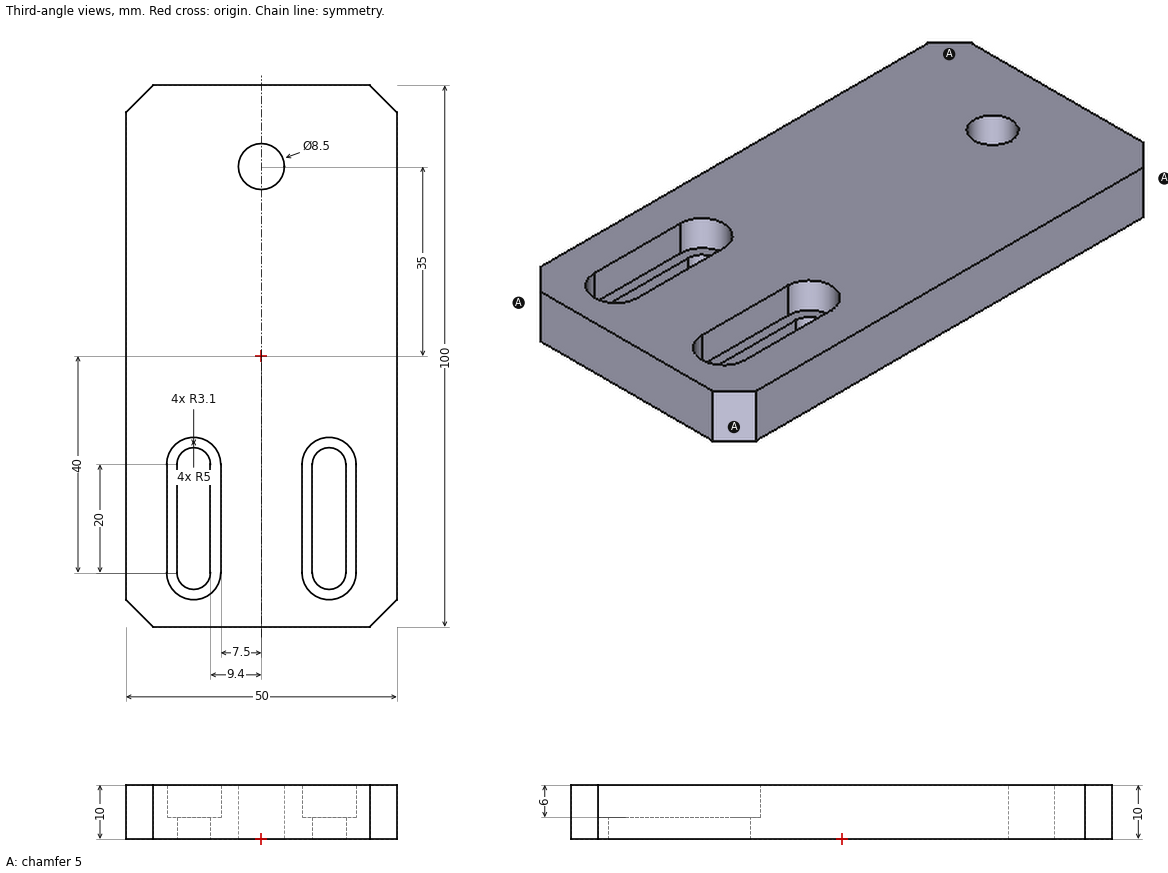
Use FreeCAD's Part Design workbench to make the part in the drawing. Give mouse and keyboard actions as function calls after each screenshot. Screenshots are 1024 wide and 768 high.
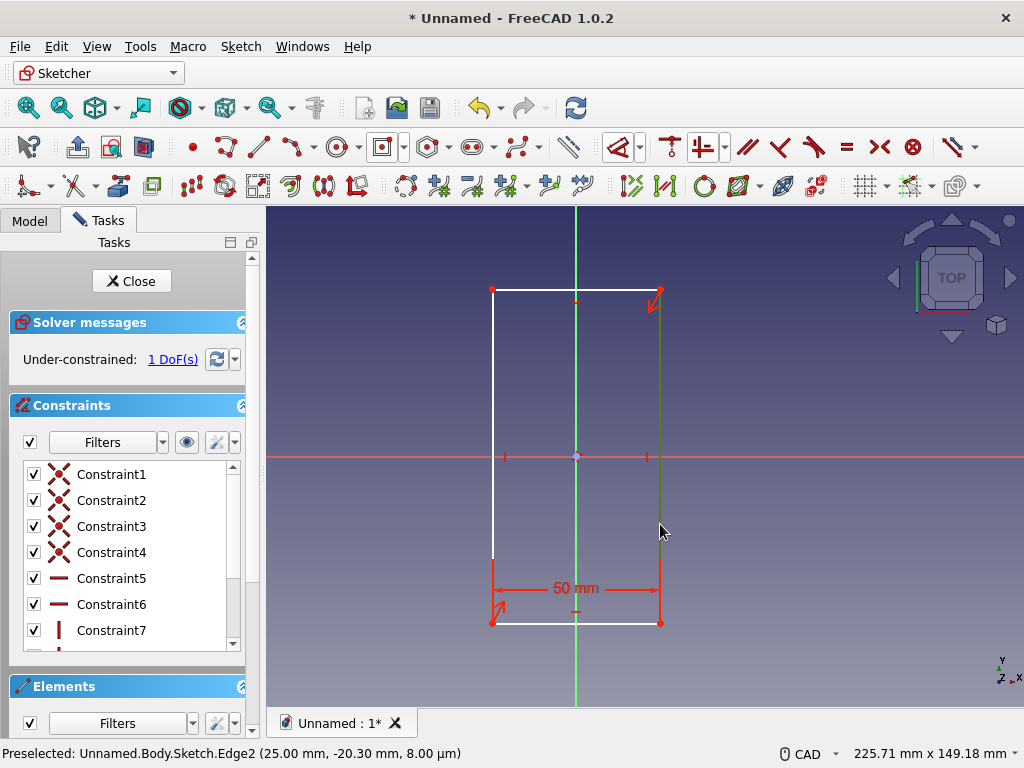
key(i)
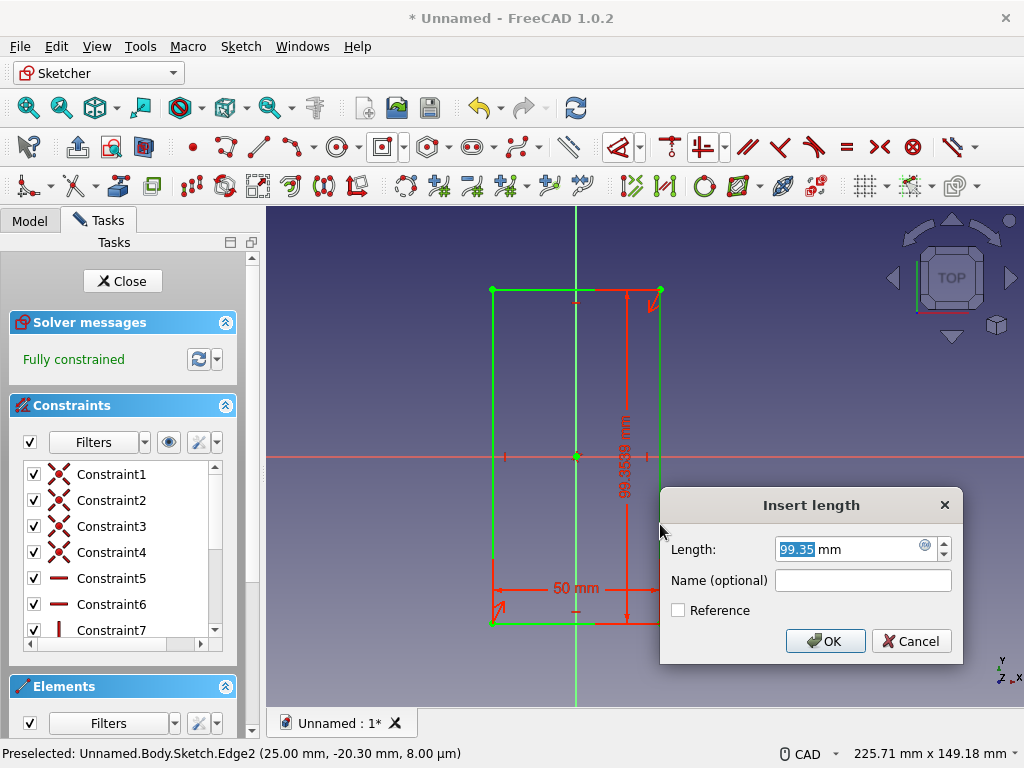
text(100)
key(Return)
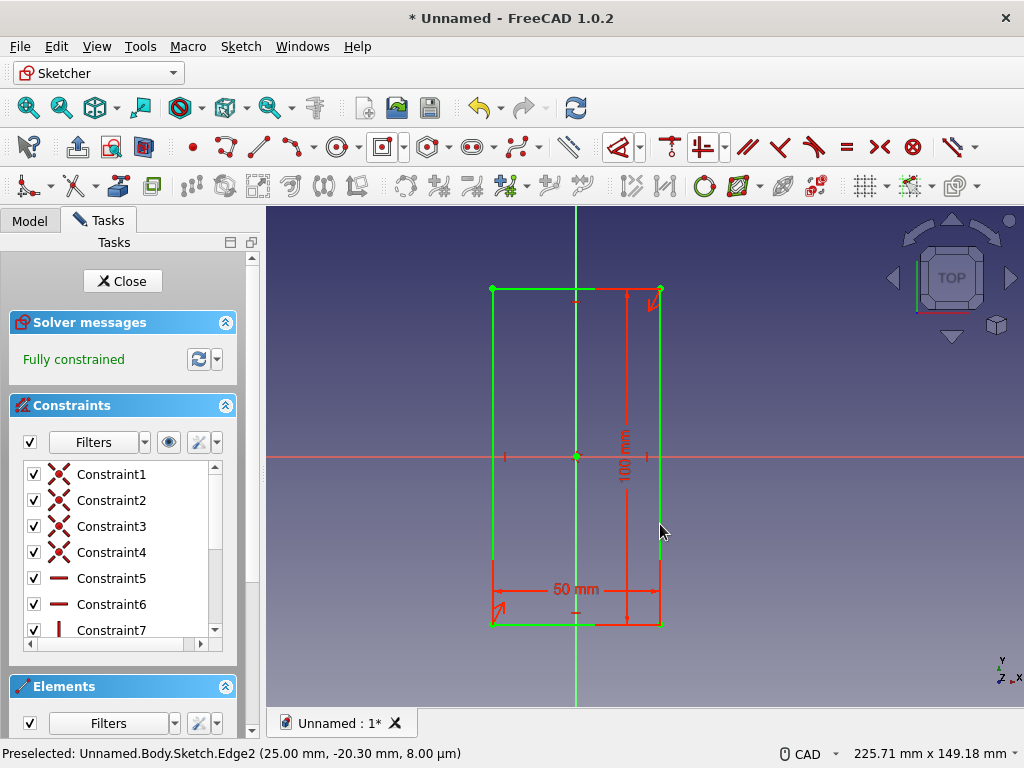
click(123, 281)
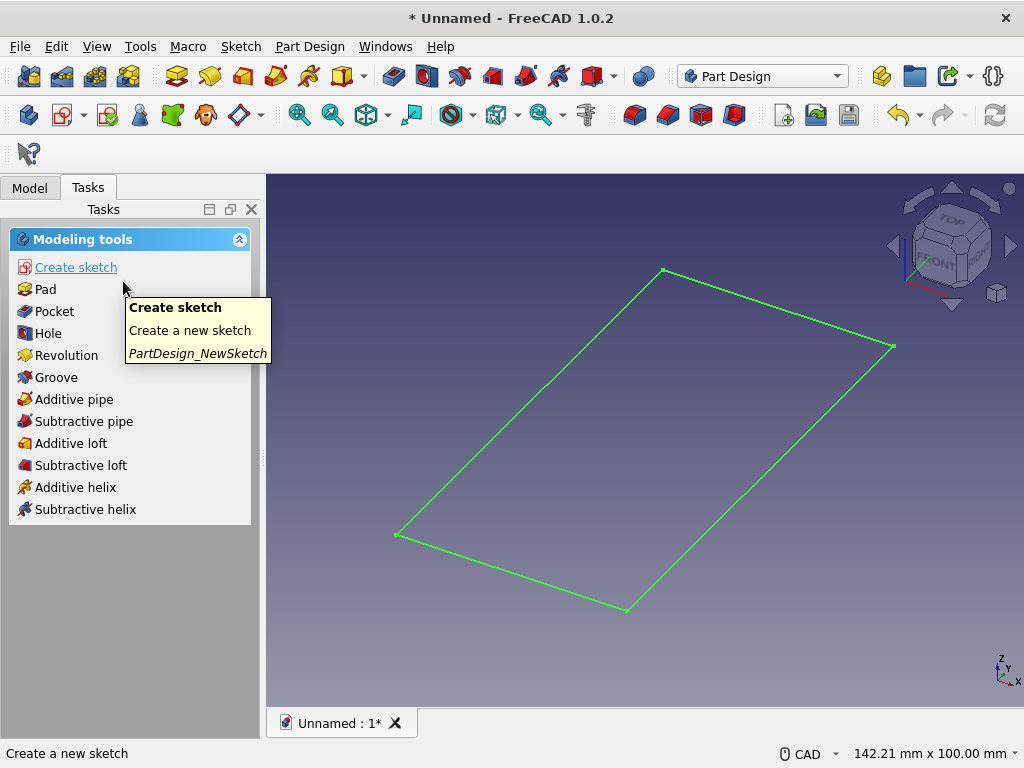
click(177, 76)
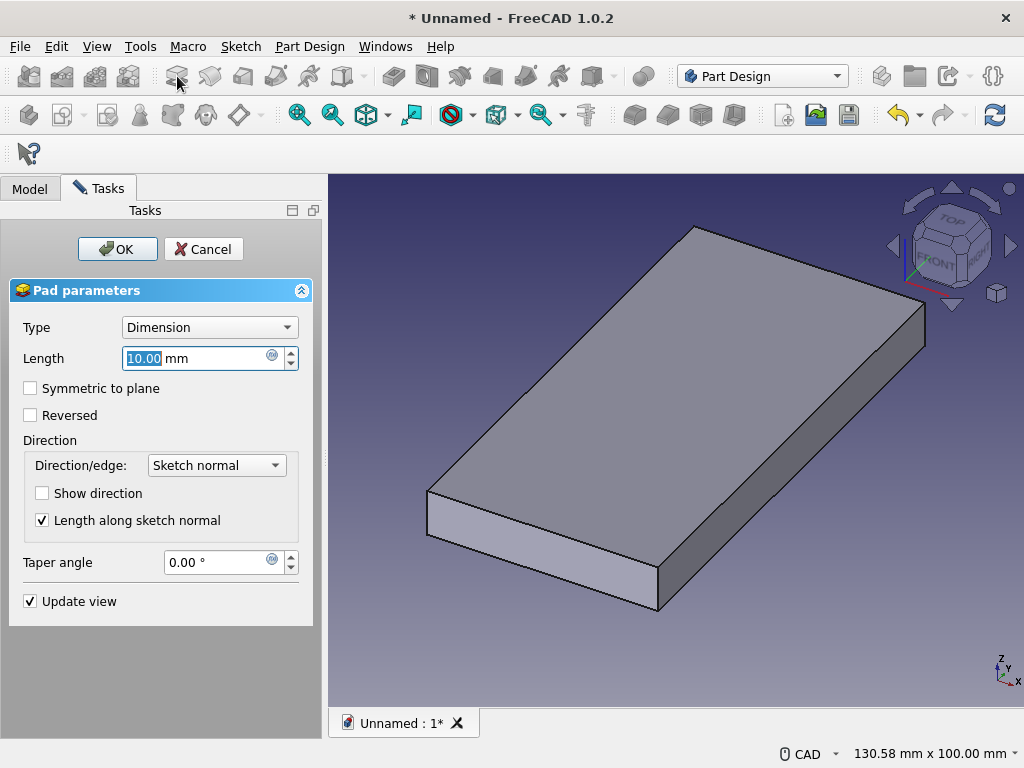
text(10)
key(Tab)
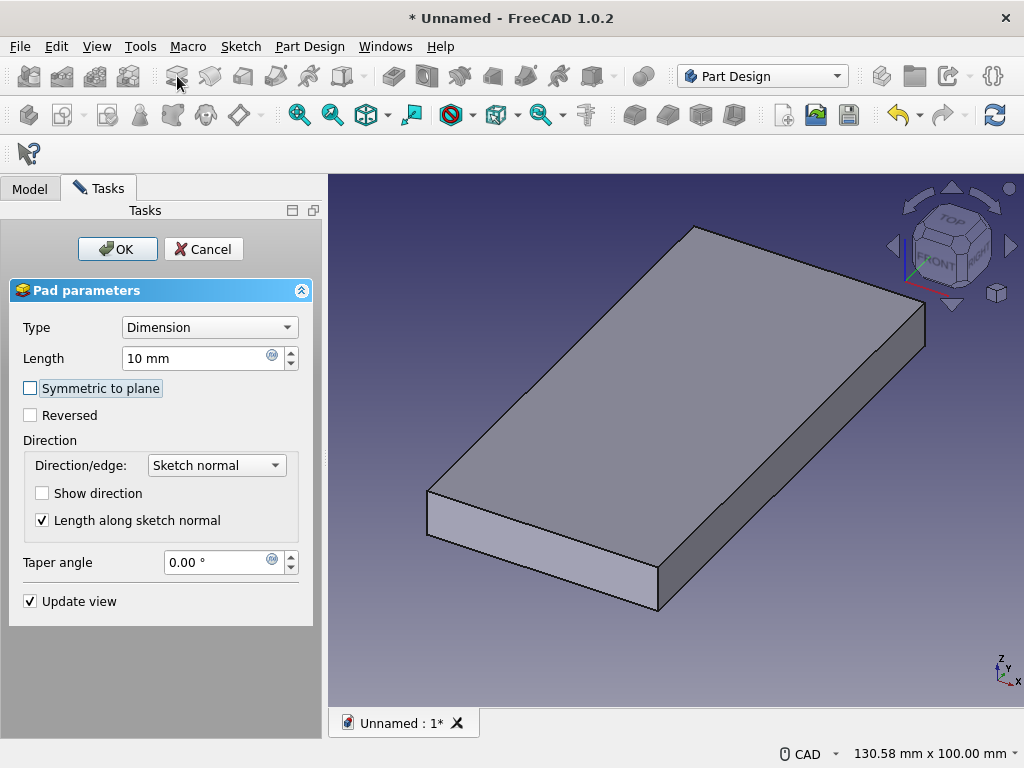
click(118, 249)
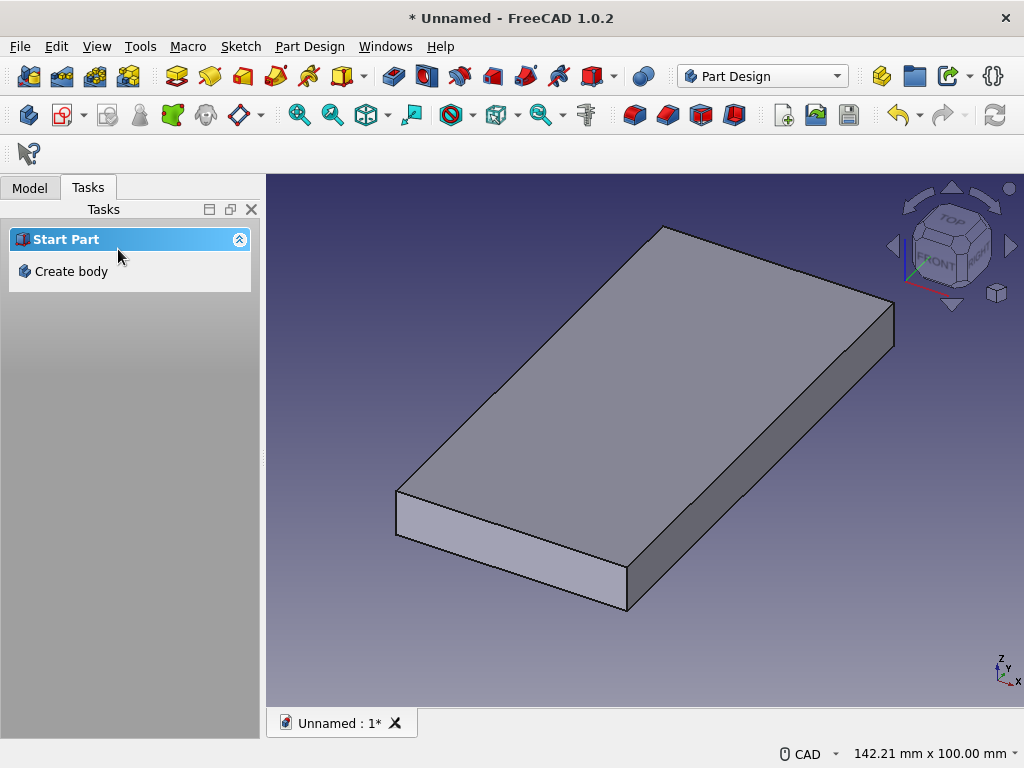
click(683, 358)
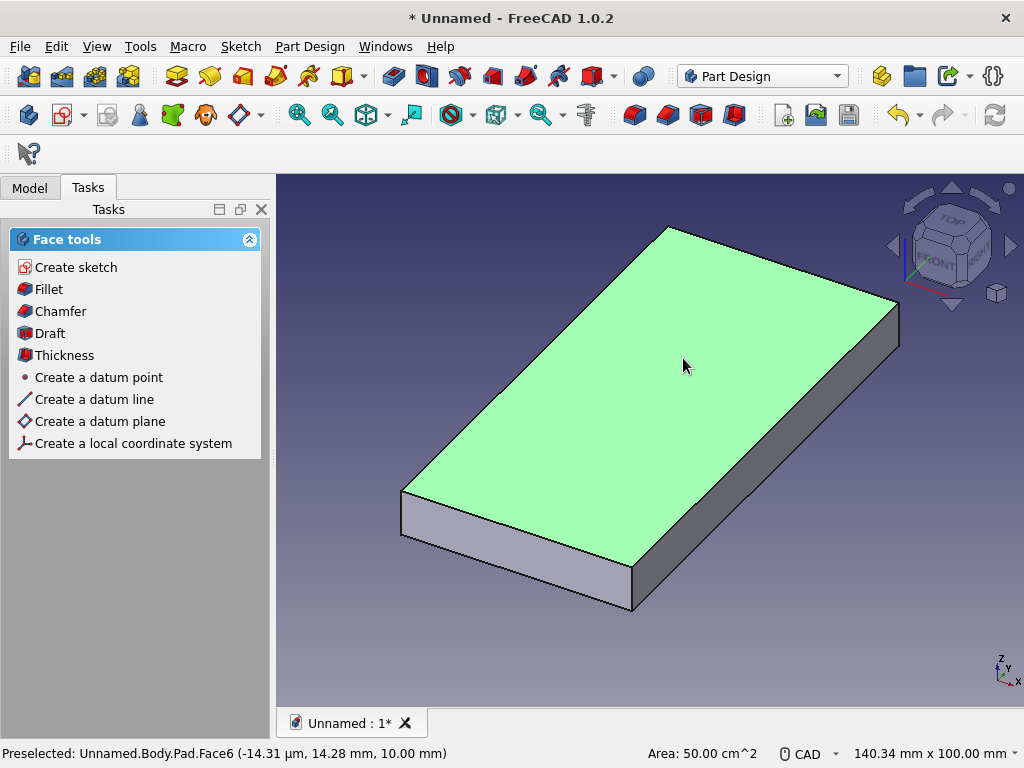
click(62, 116)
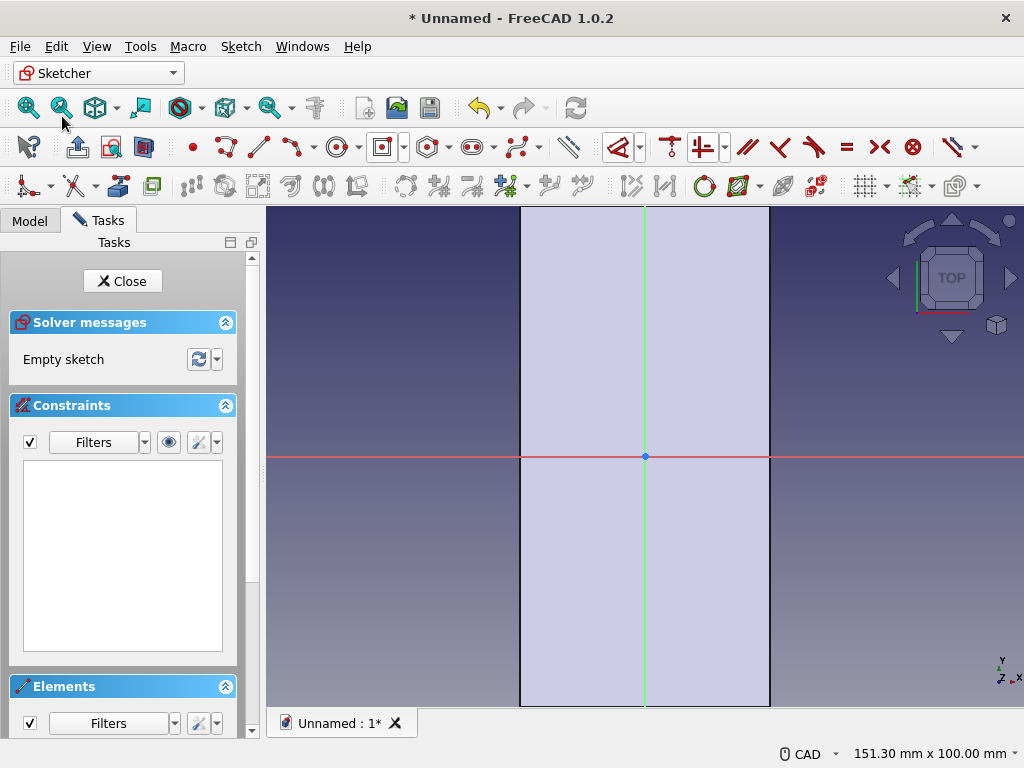
scroll(294, 234, down, 1)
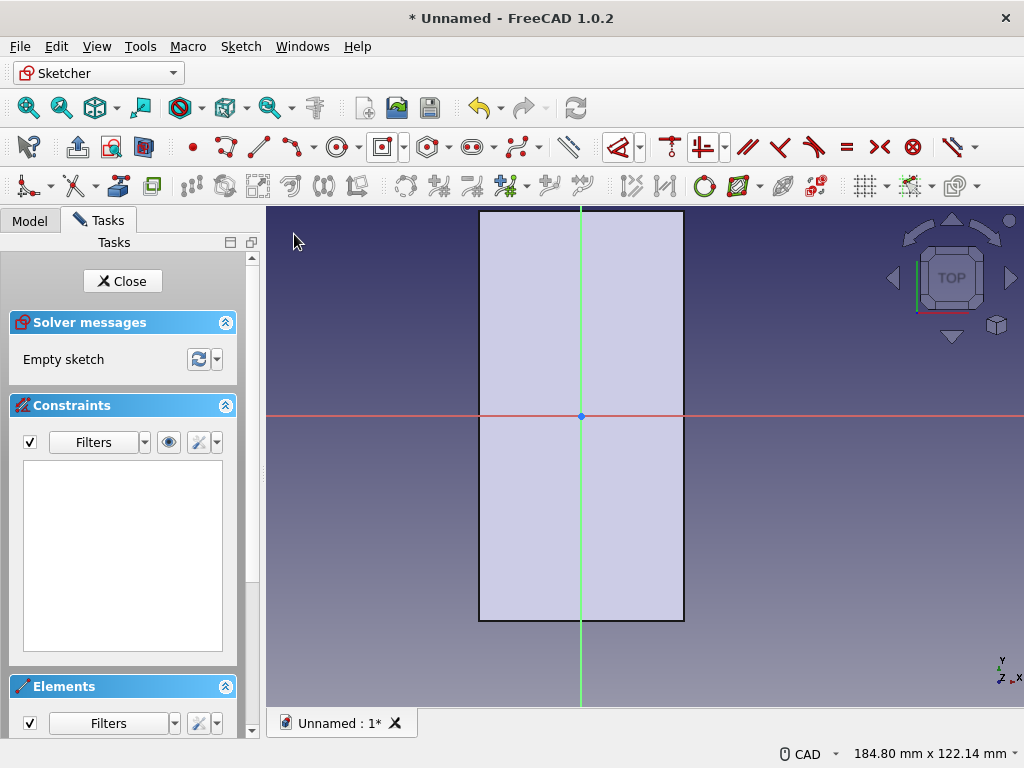
scroll(587, 563, up, 3)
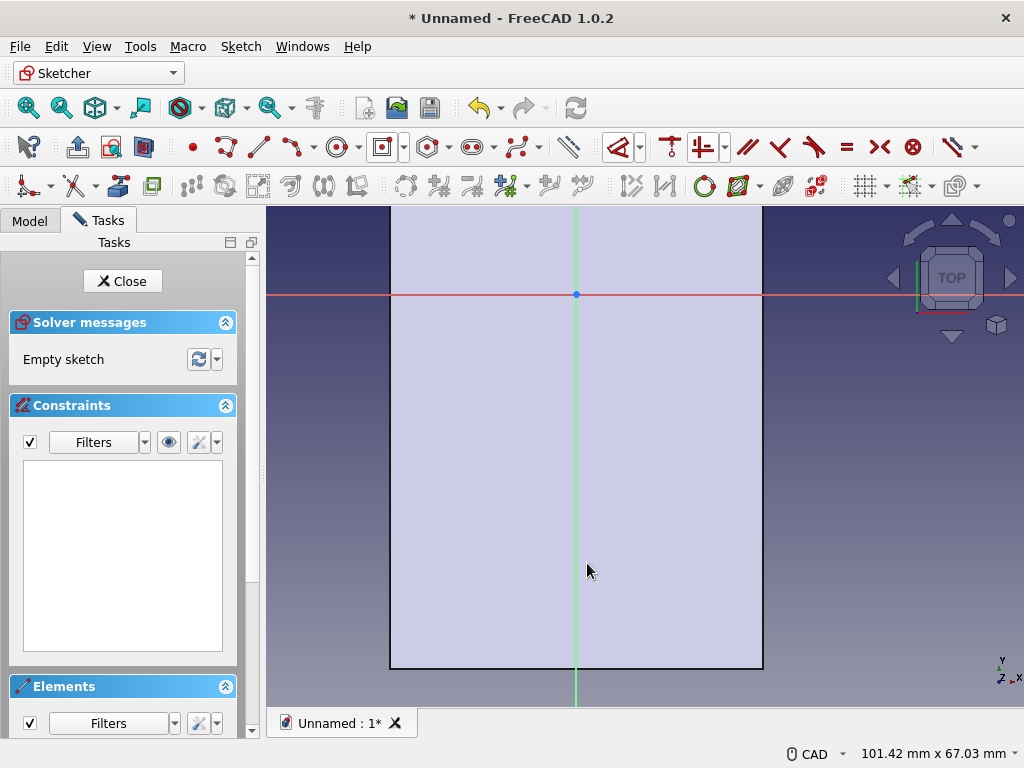
key(g)
key(s)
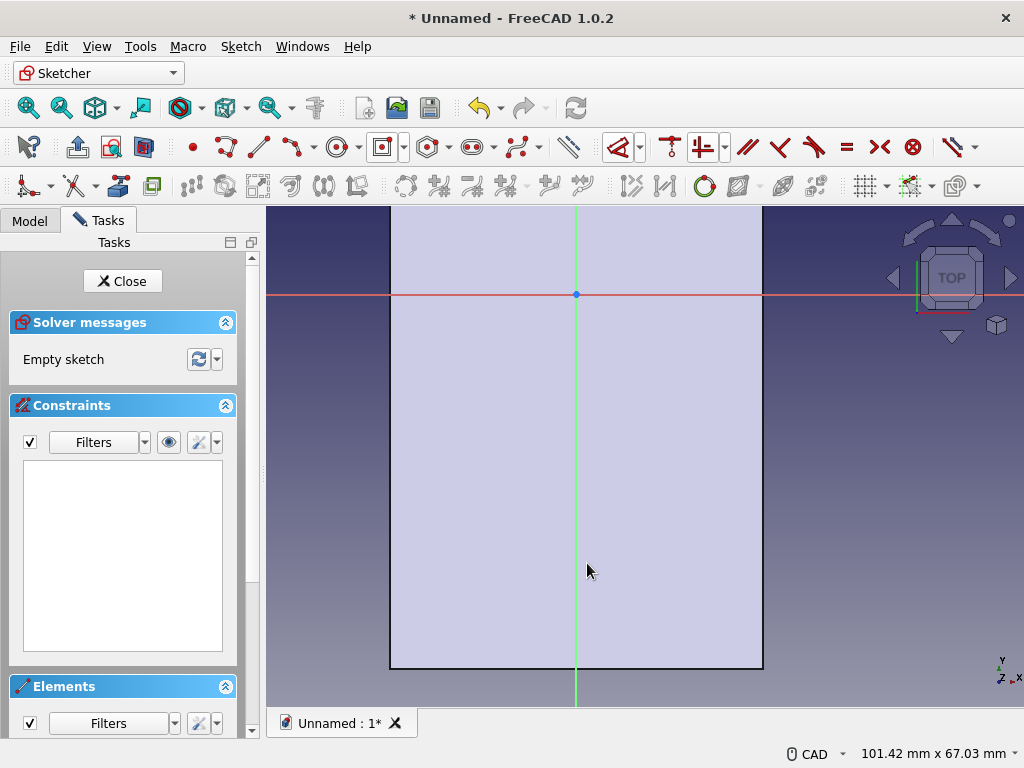
click(483, 594)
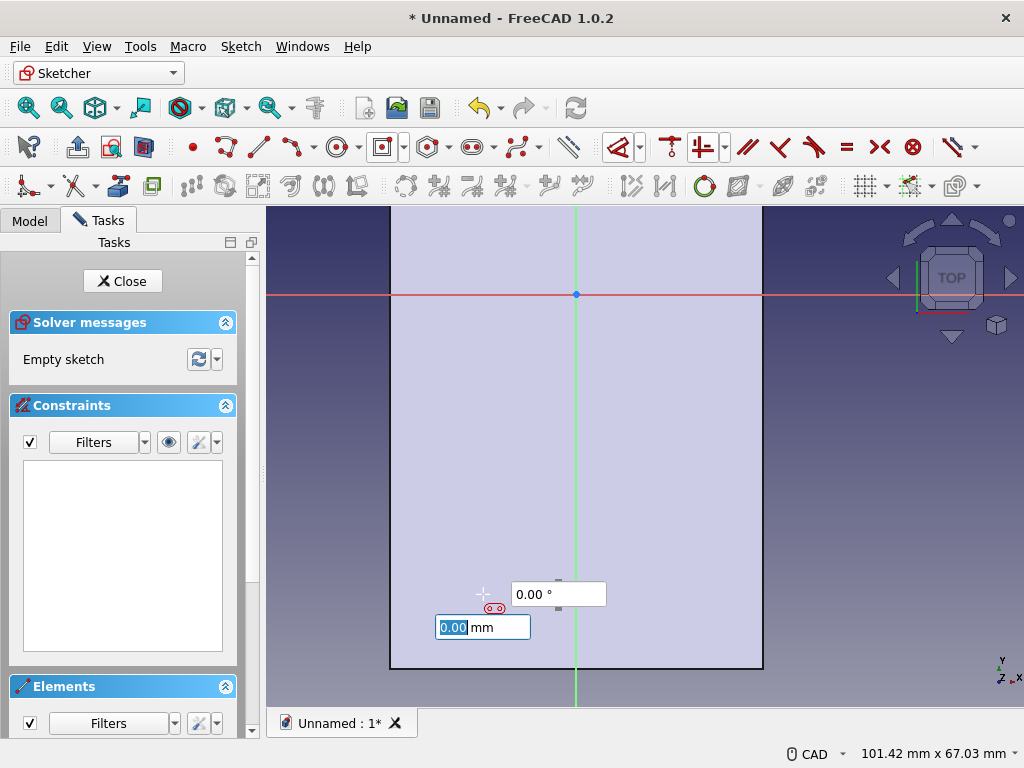
click(483, 444)